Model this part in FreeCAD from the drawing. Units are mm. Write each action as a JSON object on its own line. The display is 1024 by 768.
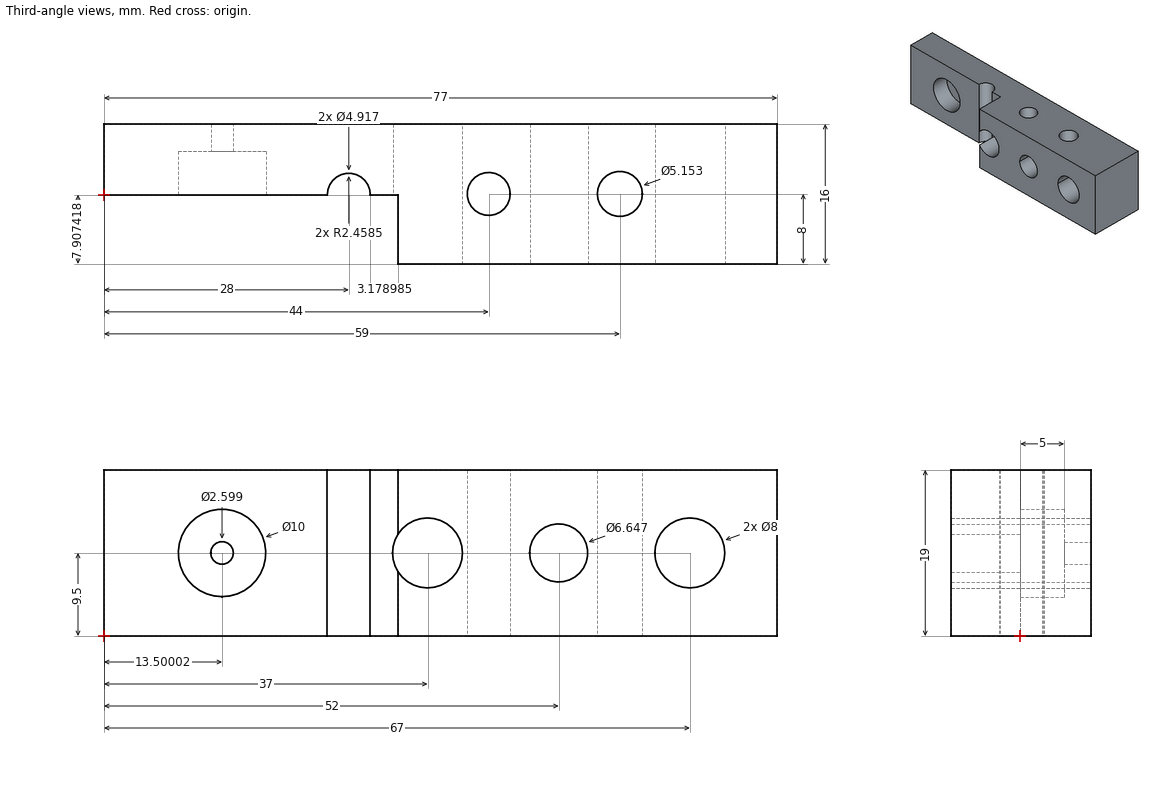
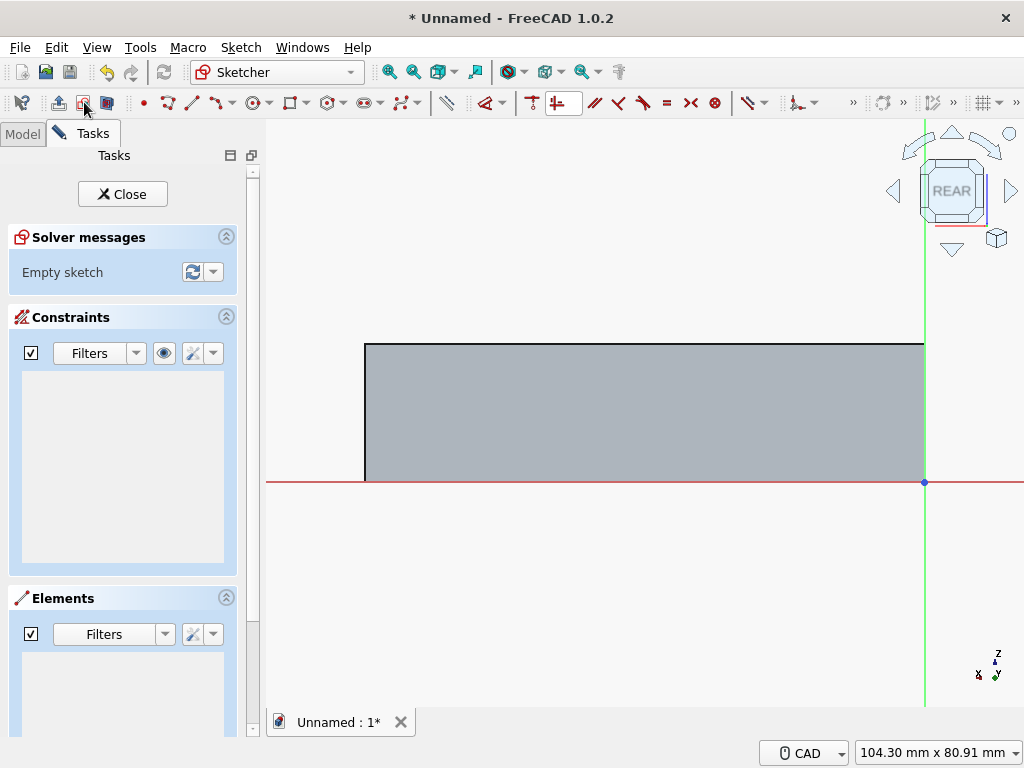
{"action": "scroll", "coordinate": [294, 323], "scroll_direction": "down", "scroll_amount": 1}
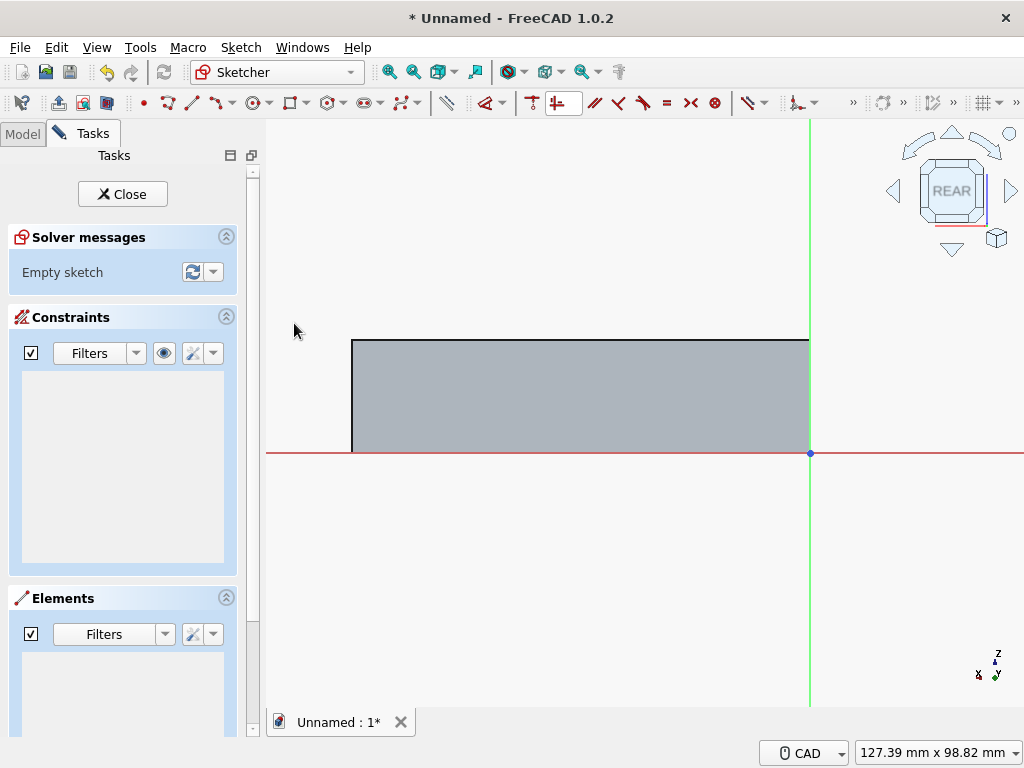
{"action": "left_click", "coordinate": [254, 104]}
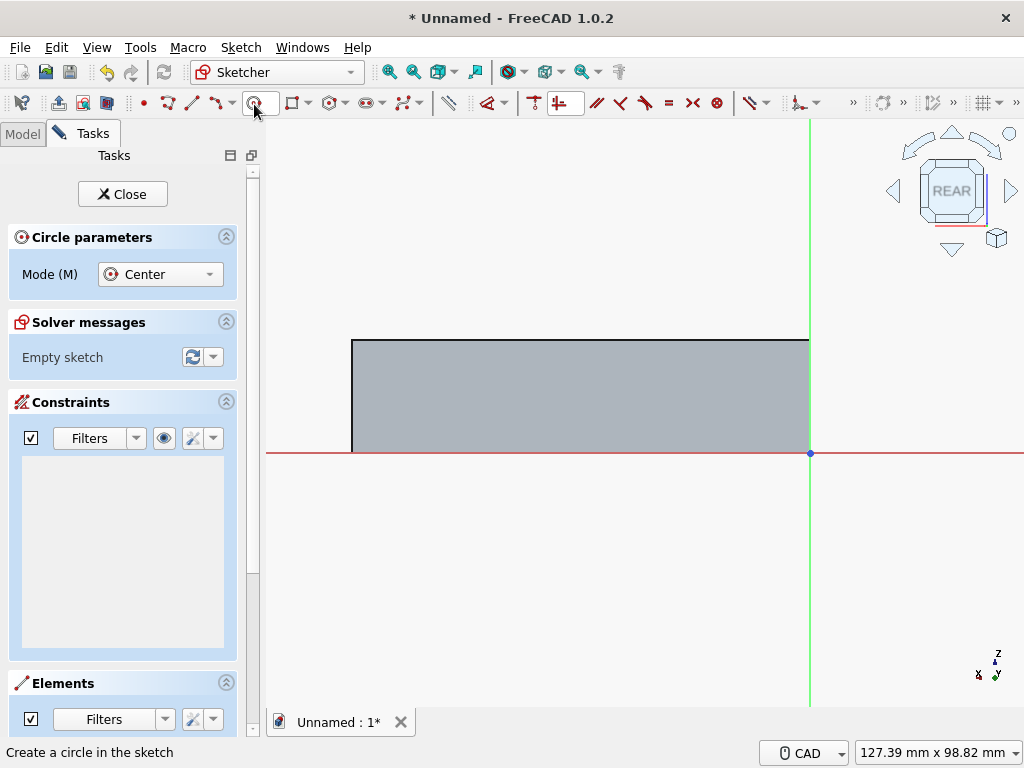
{"action": "left_click", "coordinate": [412, 397]}
{"action": "left_click", "coordinate": [429, 380]}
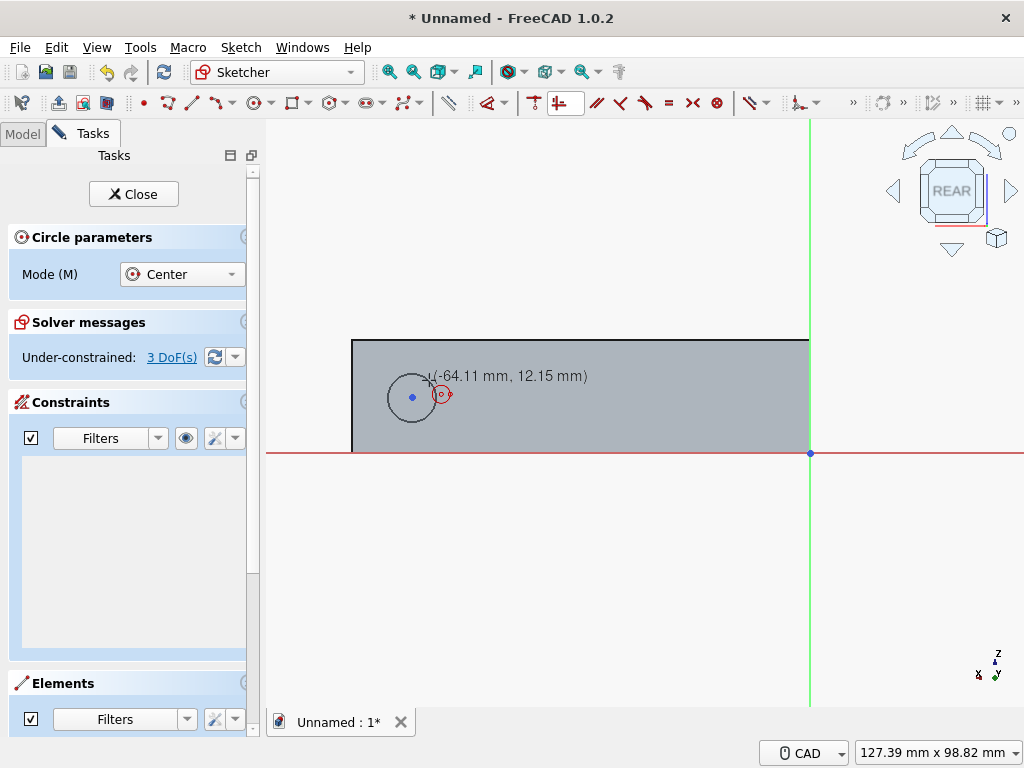
{"action": "left_click", "coordinate": [501, 397]}
{"action": "left_click", "coordinate": [515, 383]}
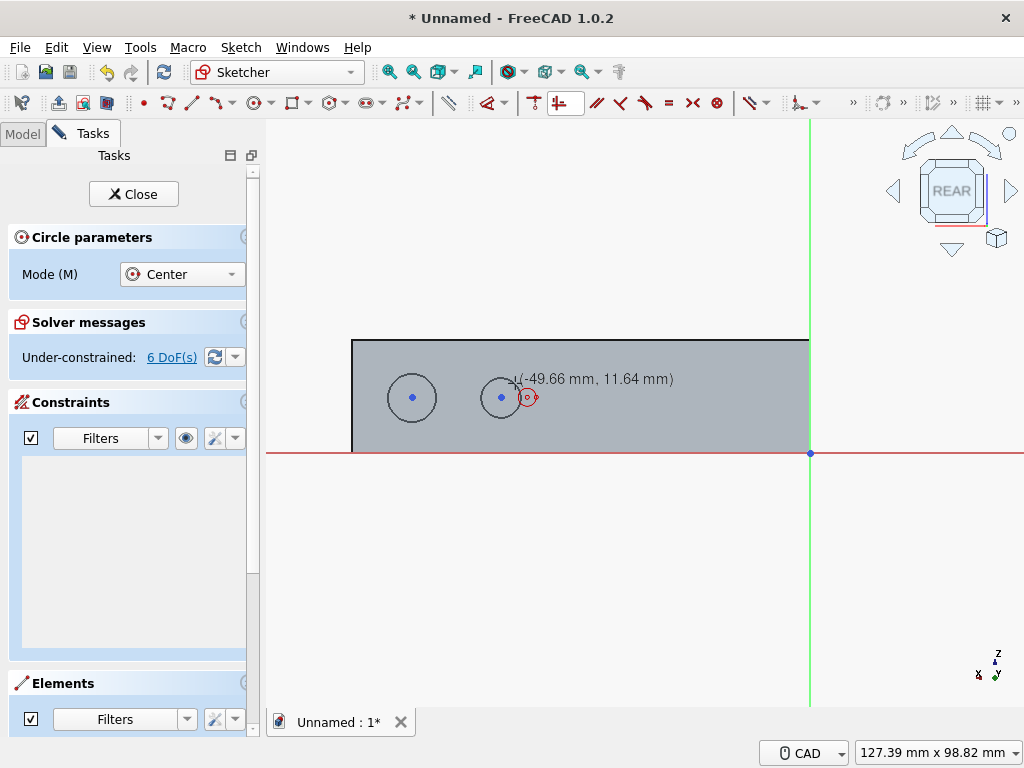
{"action": "left_click", "coordinate": [590, 397]}
{"action": "left_click", "coordinate": [607, 380]}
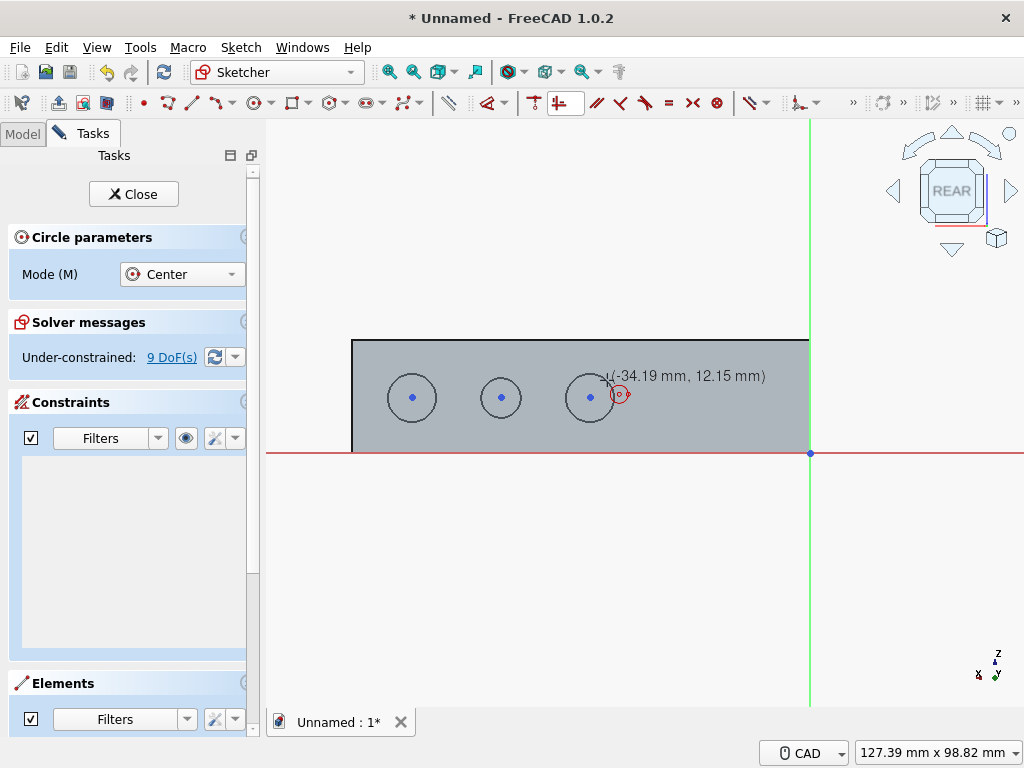
{"action": "scroll", "coordinate": [730, 397], "scroll_direction": "up", "scroll_amount": 6}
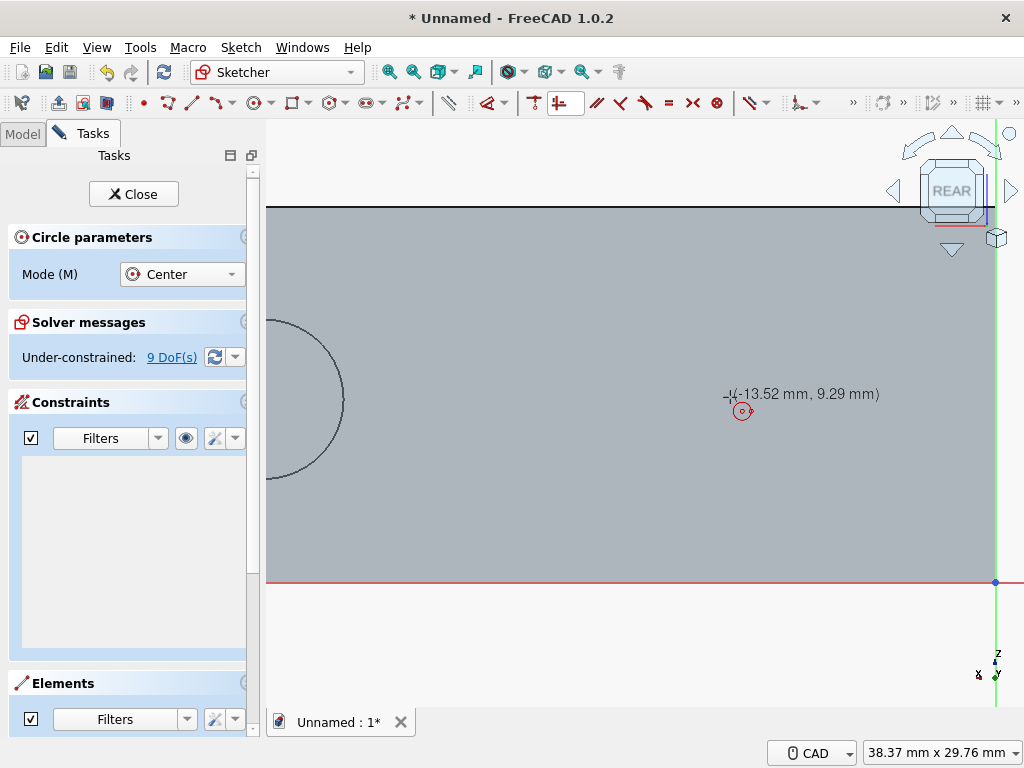
{"action": "left_click", "coordinate": [729, 395]}
{"action": "left_click", "coordinate": [747, 377]}
{"action": "key", "text": "Escape"}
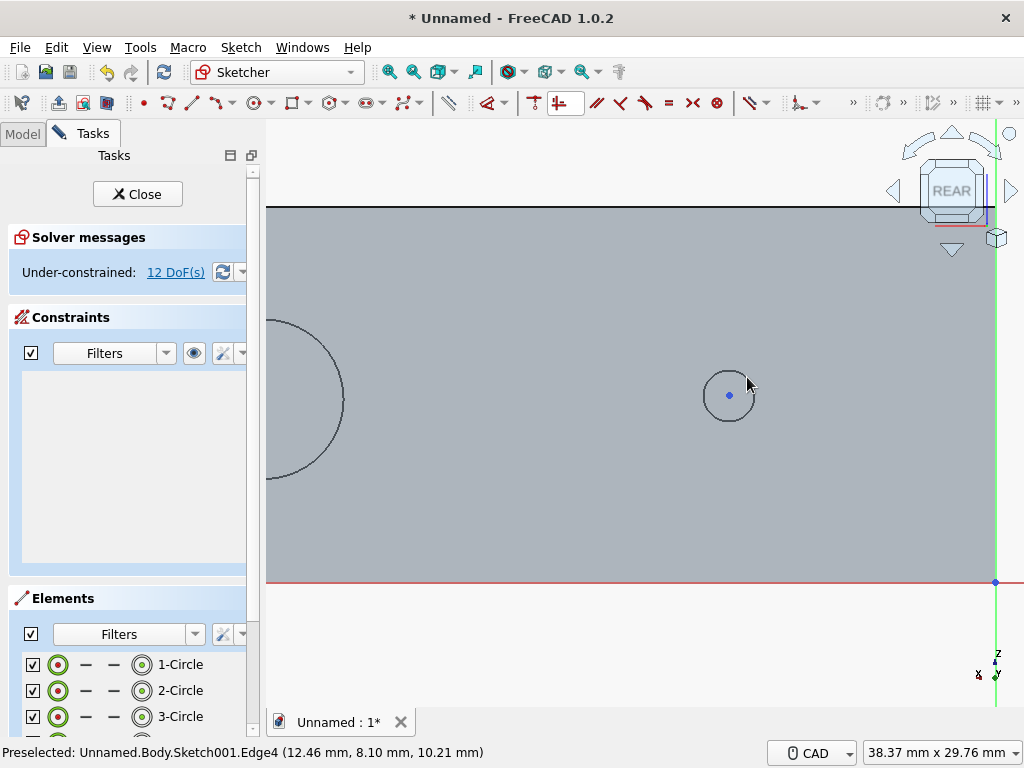
{"action": "scroll", "coordinate": [698, 397], "scroll_direction": "down", "scroll_amount": 6}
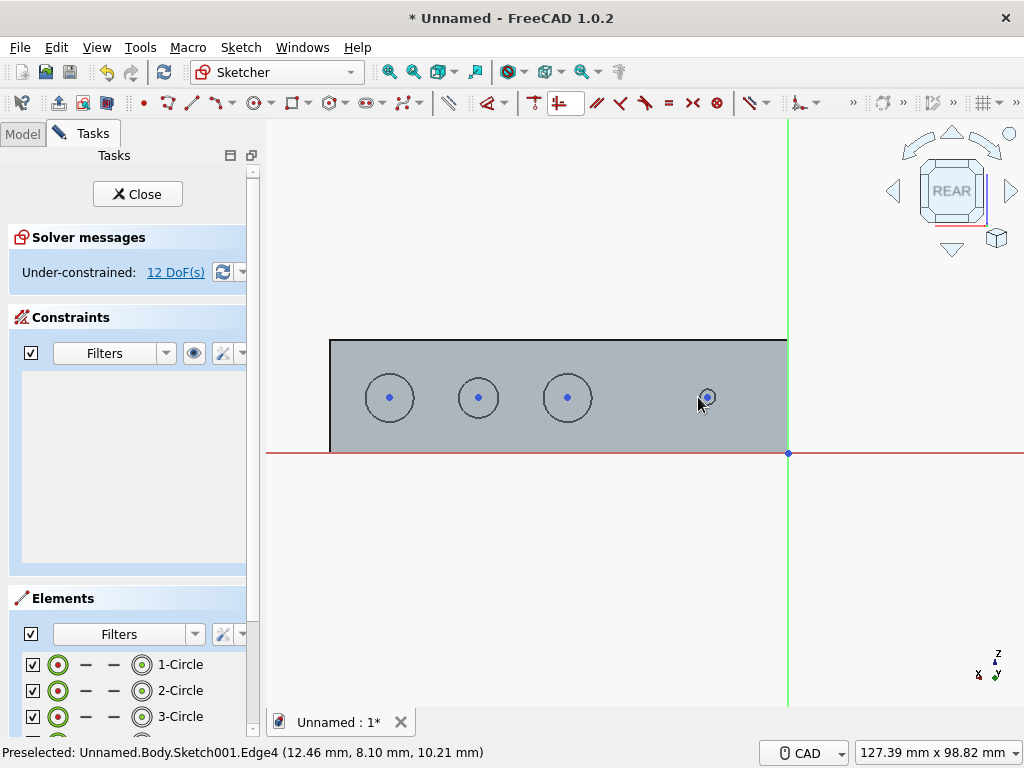
{"action": "left_click", "coordinate": [407, 381]}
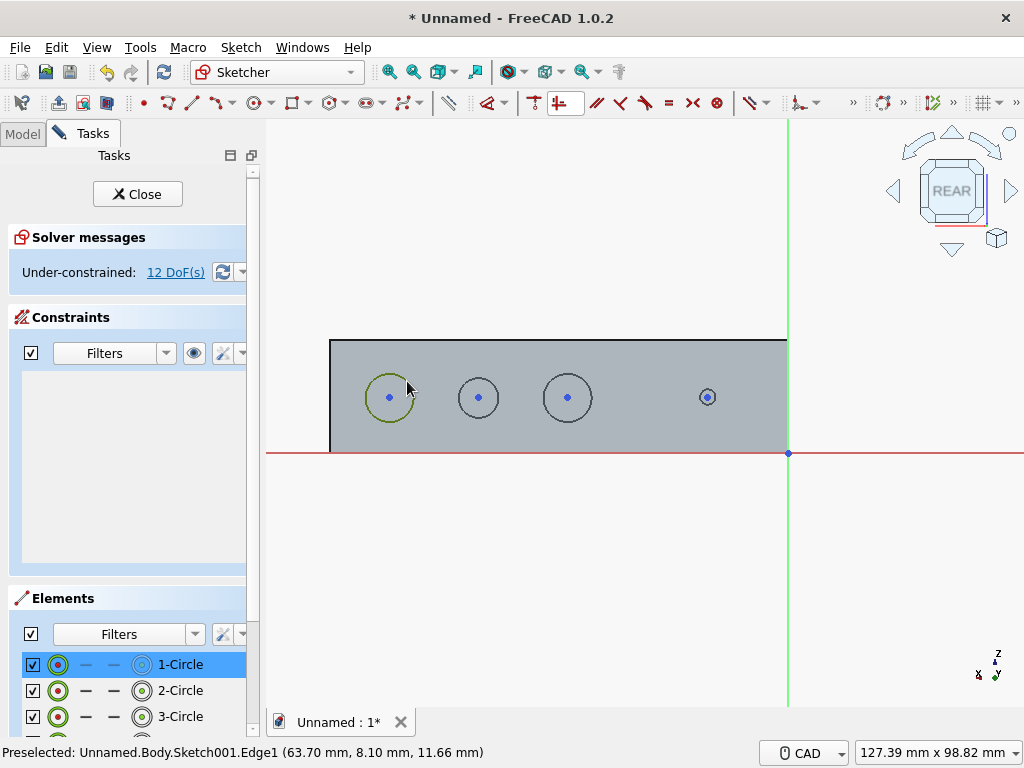
{"action": "left_click", "coordinate": [585, 381]}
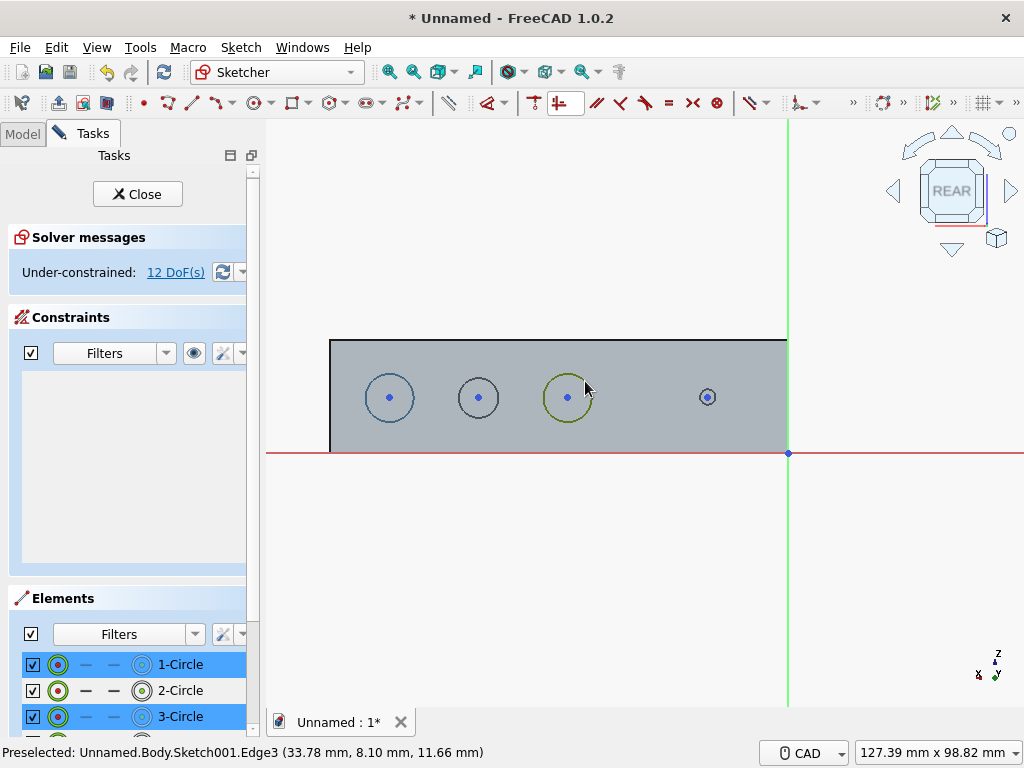
{"action": "left_click", "coordinate": [670, 104]}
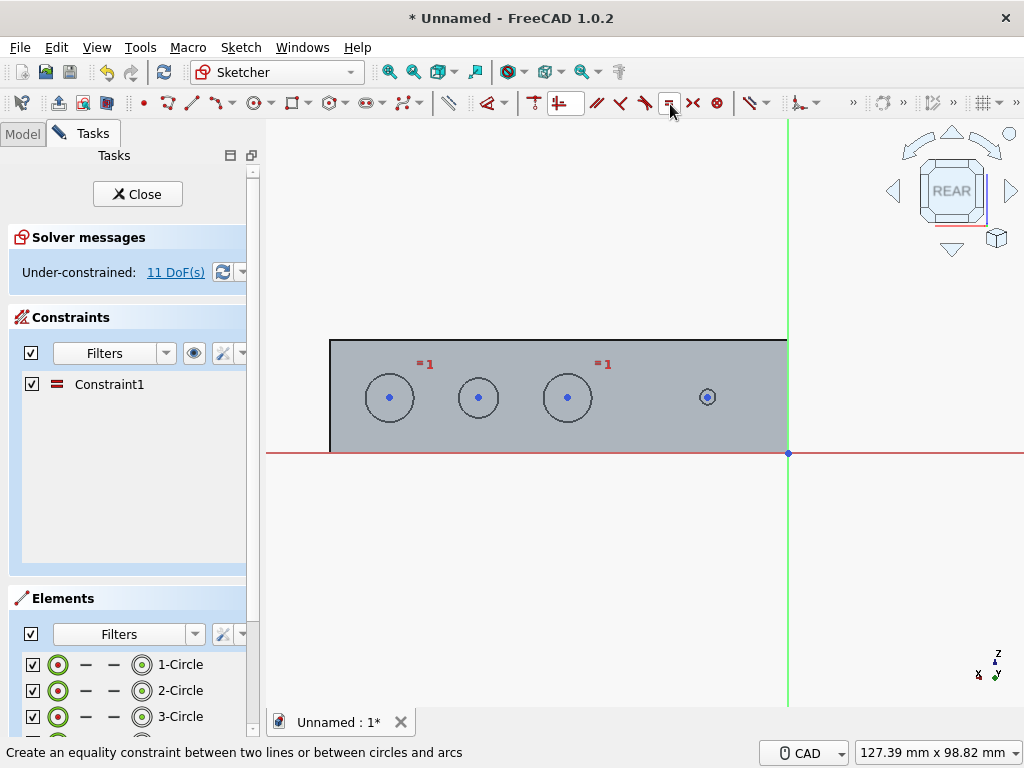
{"action": "left_click", "coordinate": [390, 398]}